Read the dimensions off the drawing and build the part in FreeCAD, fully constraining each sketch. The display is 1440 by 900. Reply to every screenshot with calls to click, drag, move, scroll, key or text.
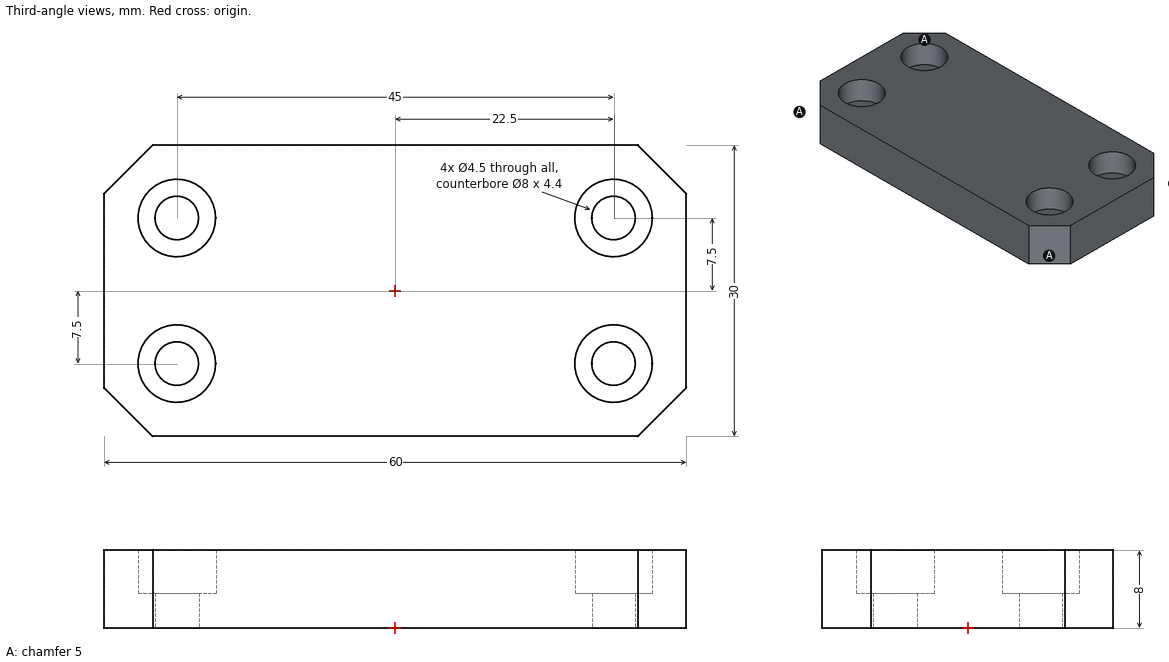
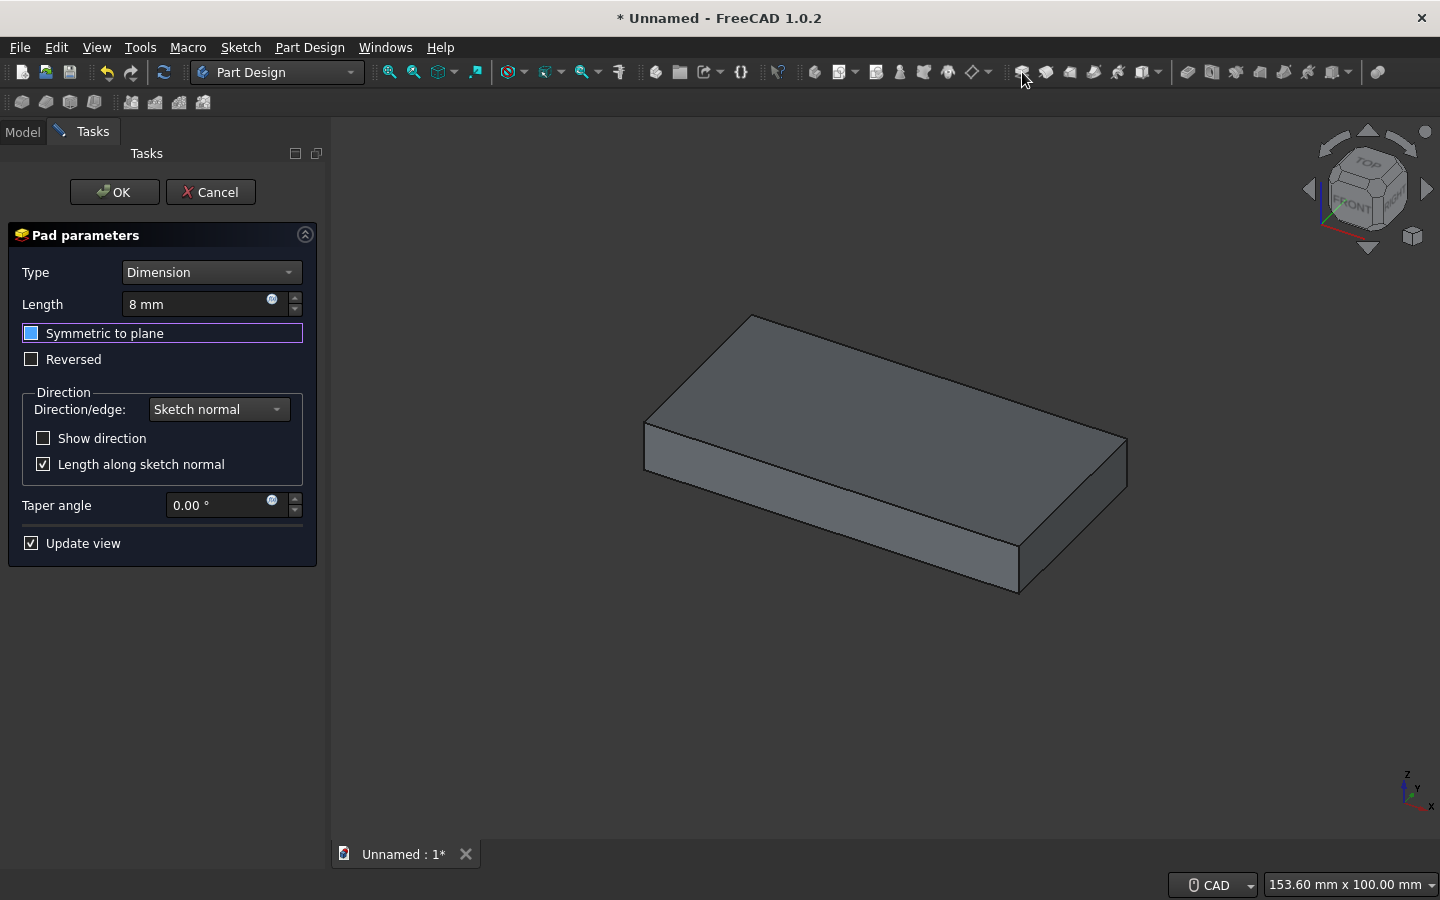
click(115, 192)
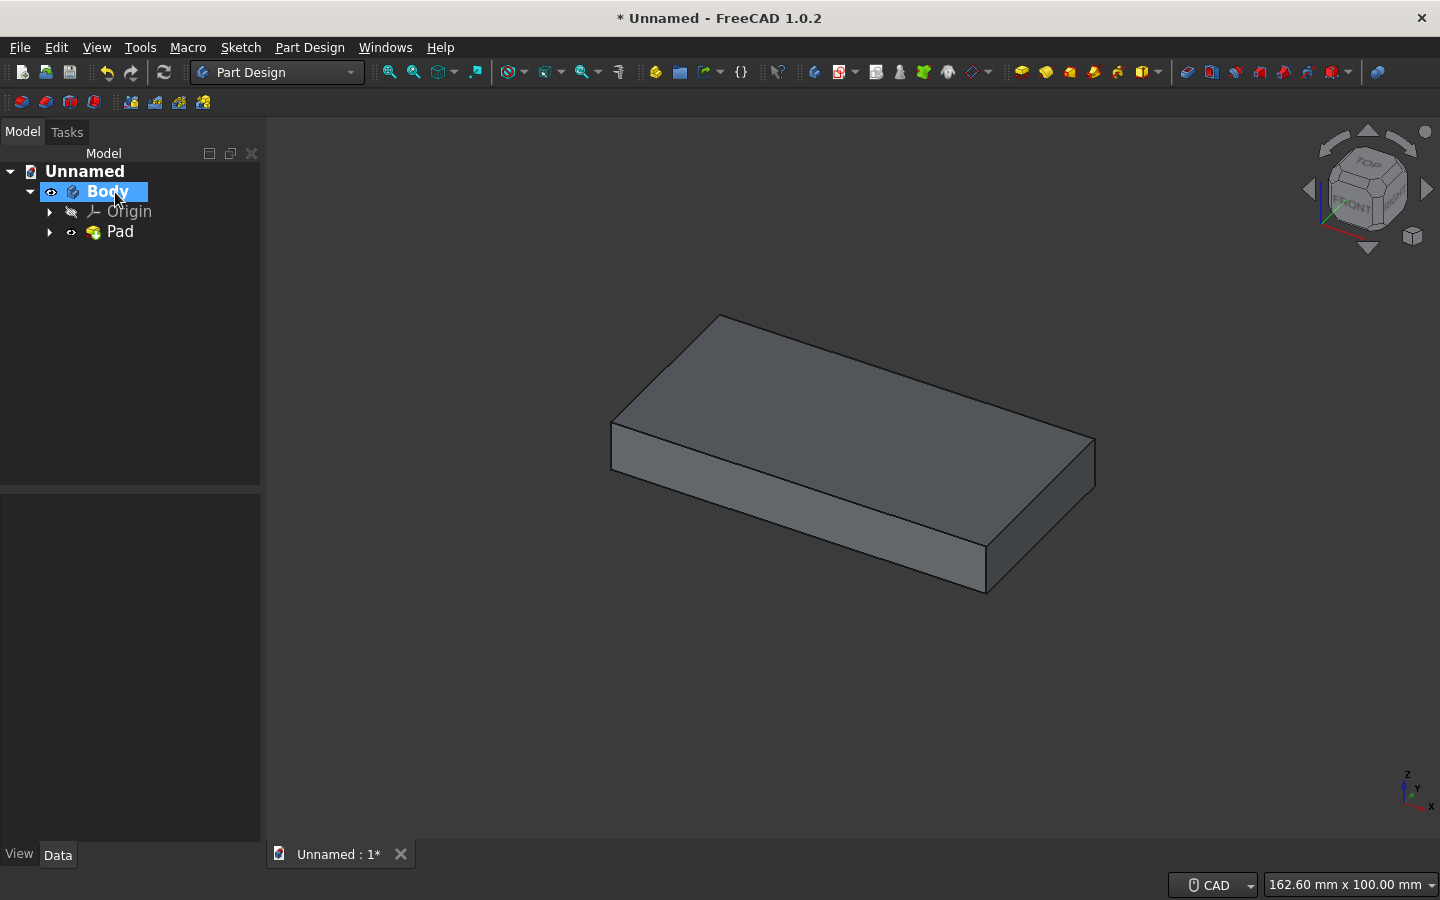
click(390, 72)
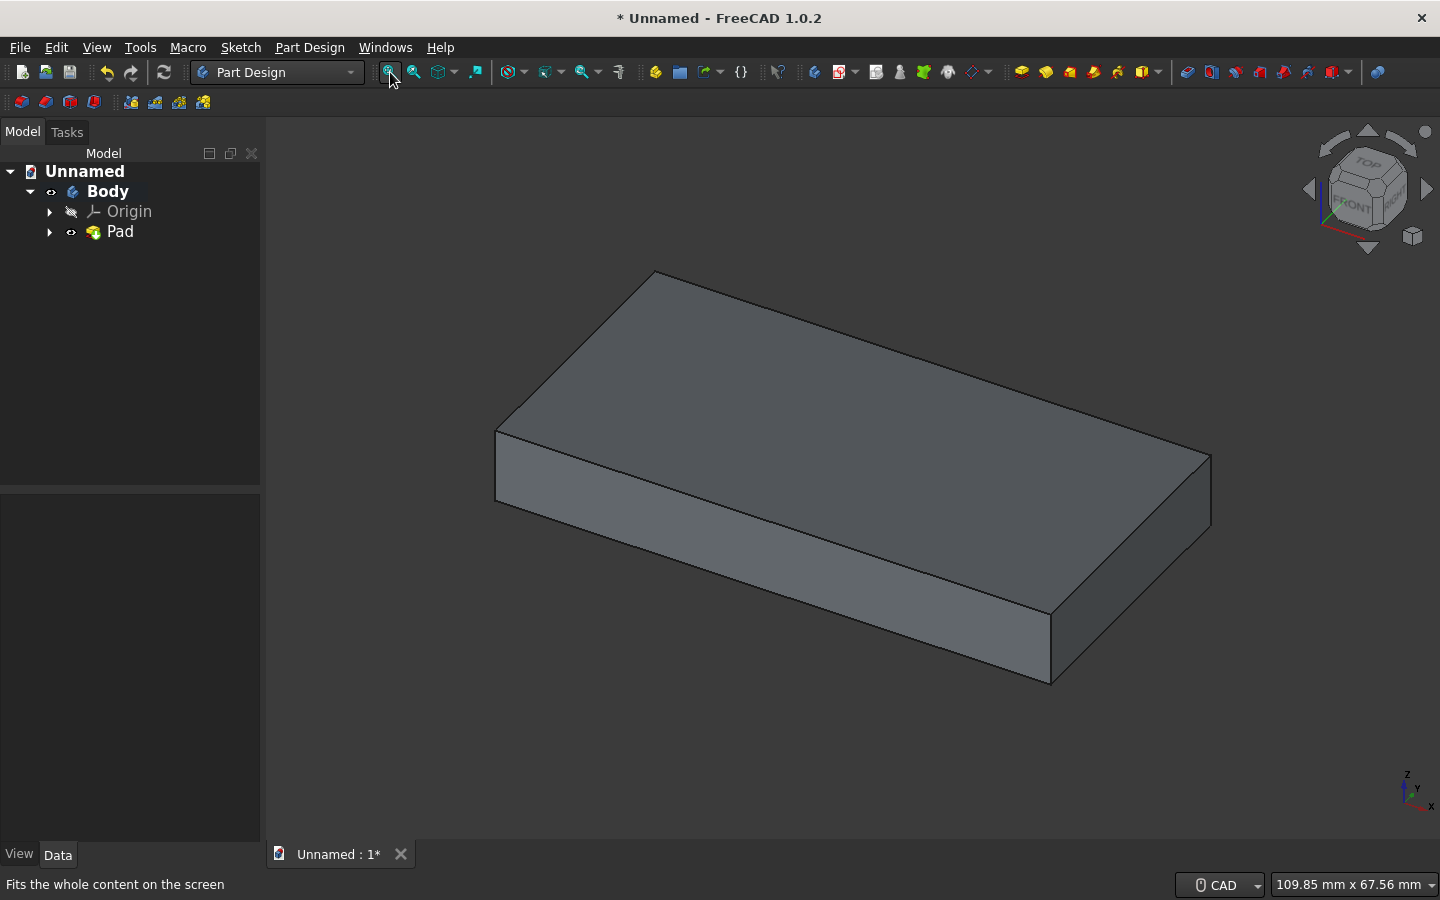
click(932, 468)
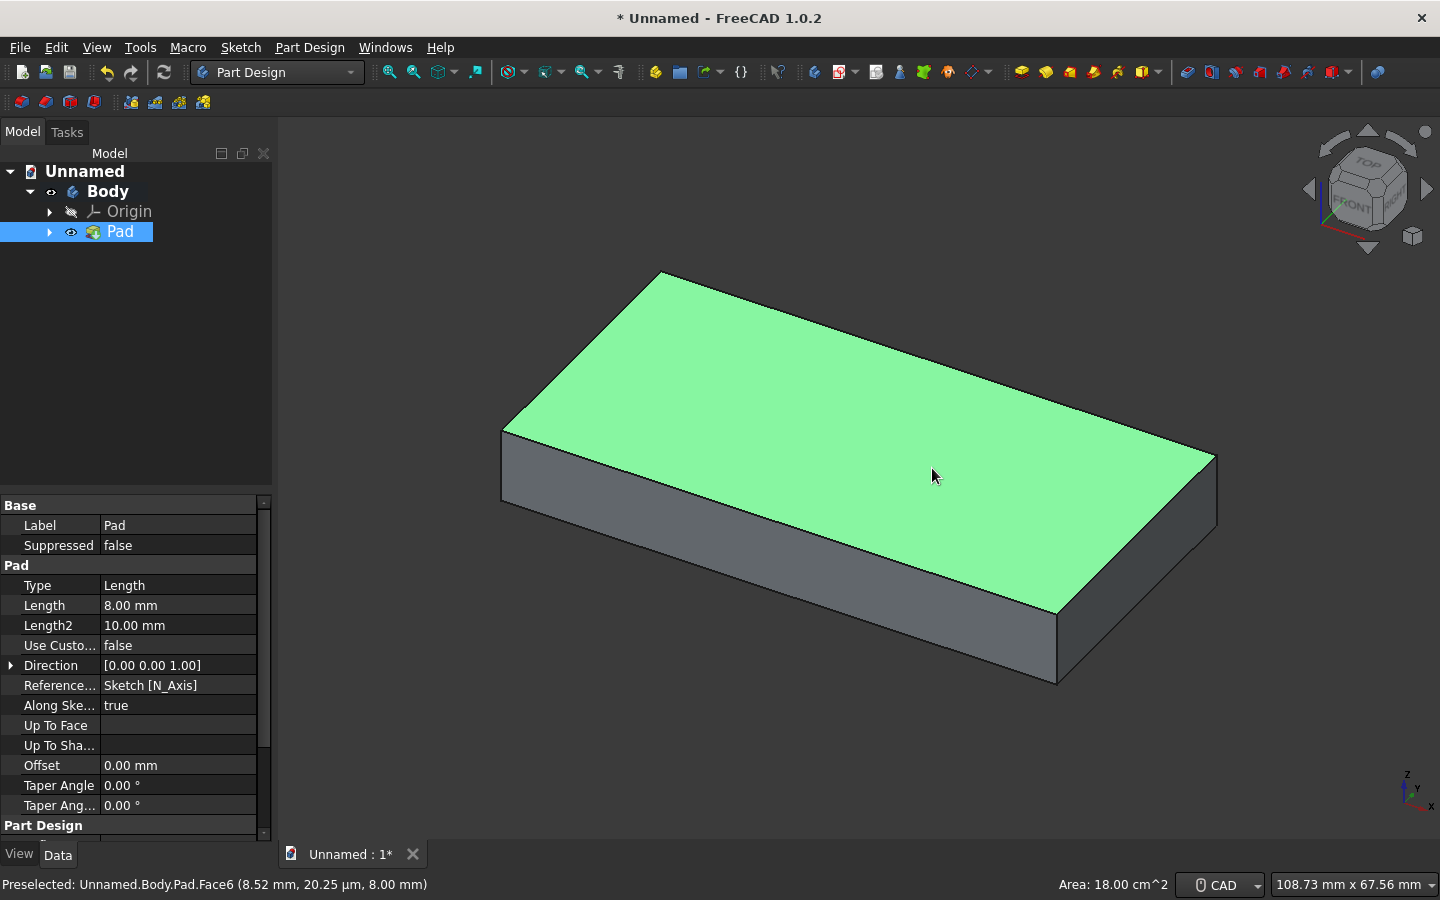
click(840, 72)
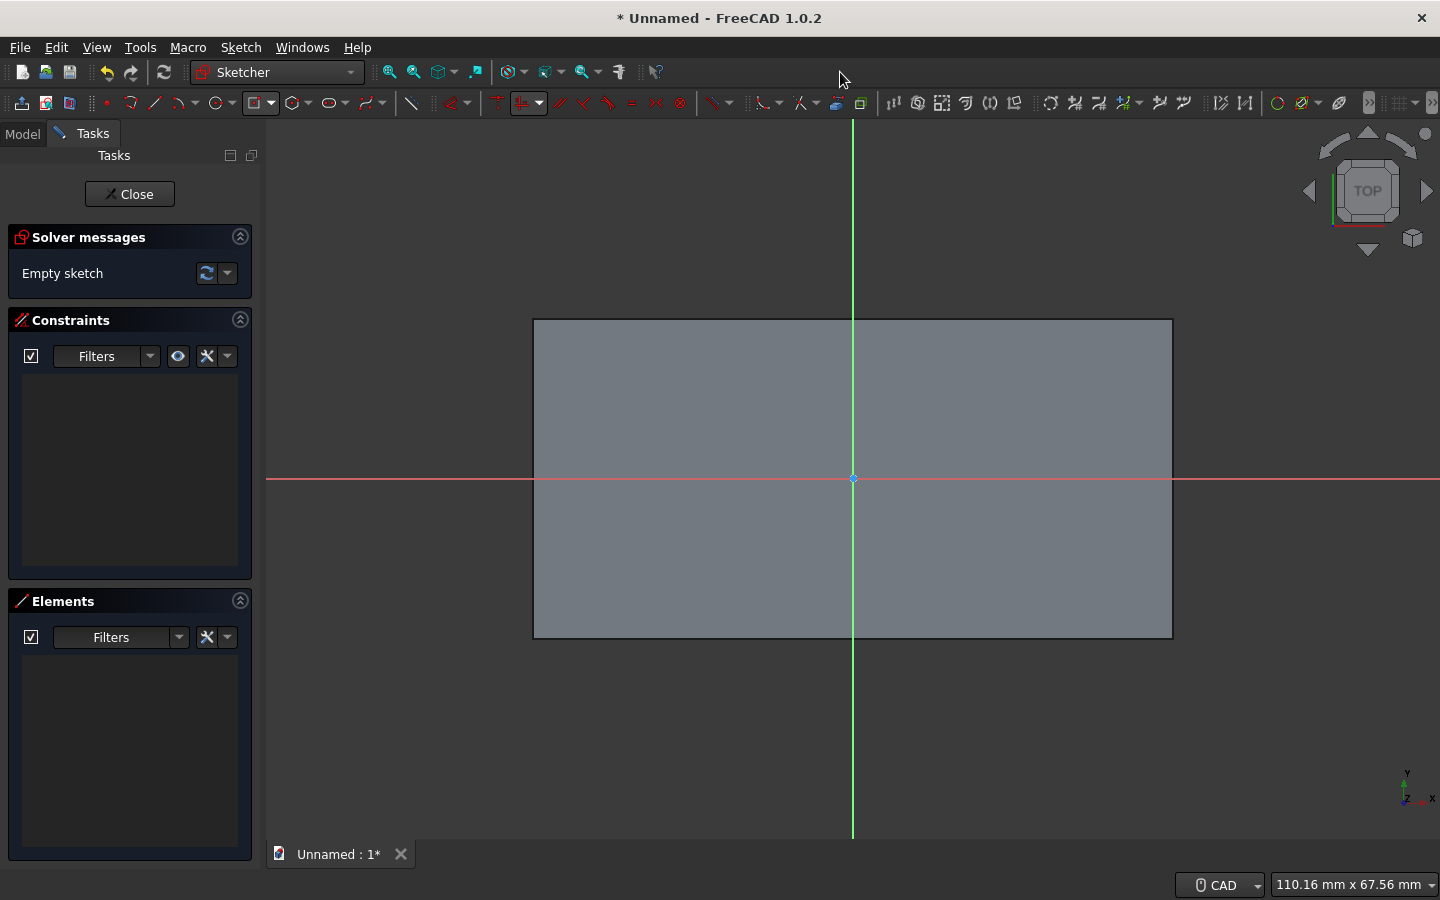
click(216, 104)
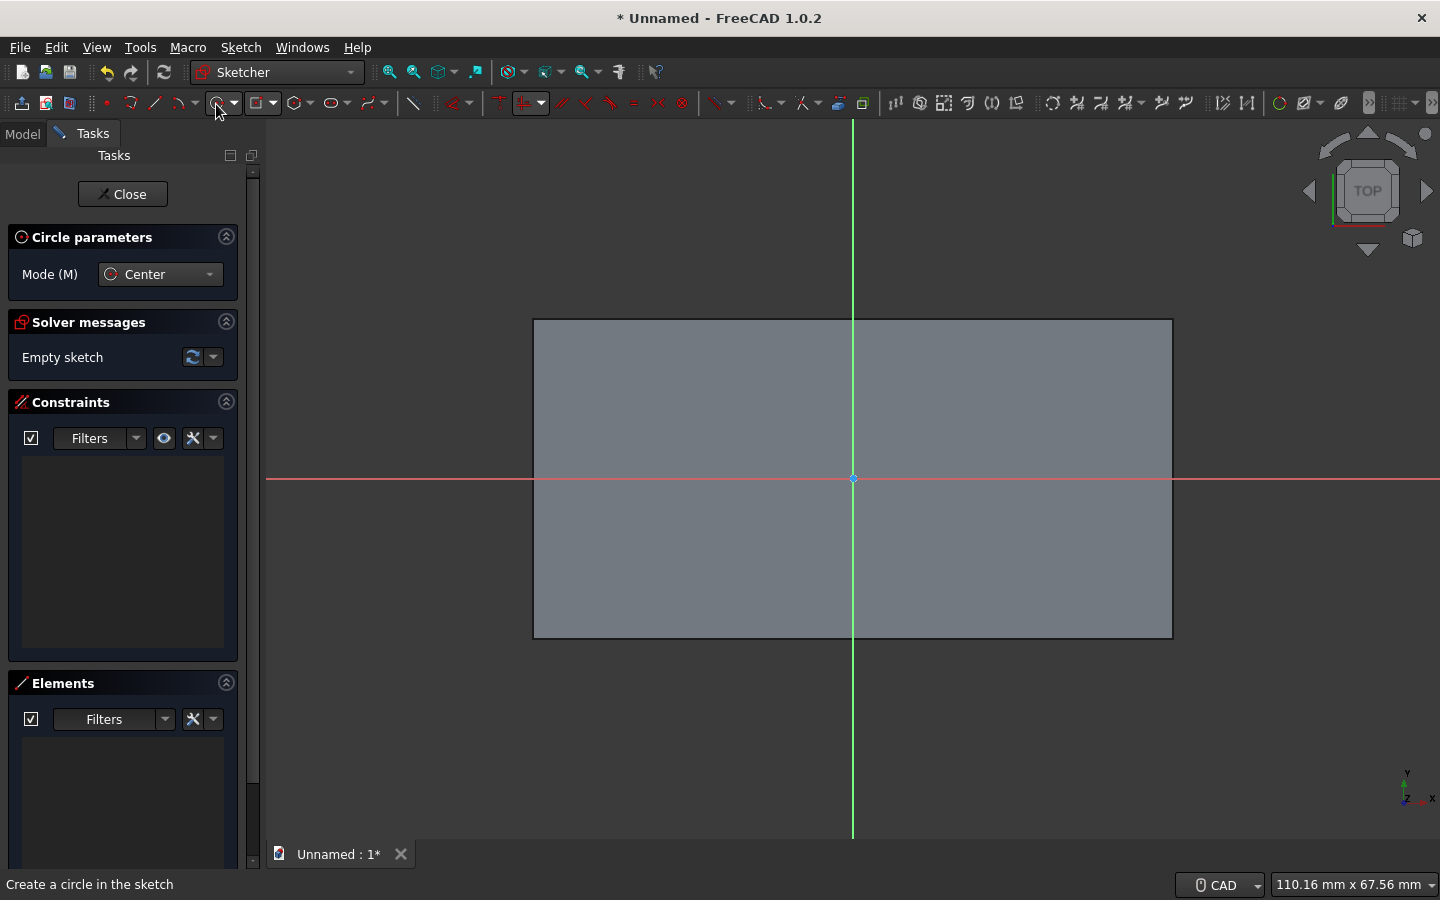
click(1093, 399)
click(1110, 382)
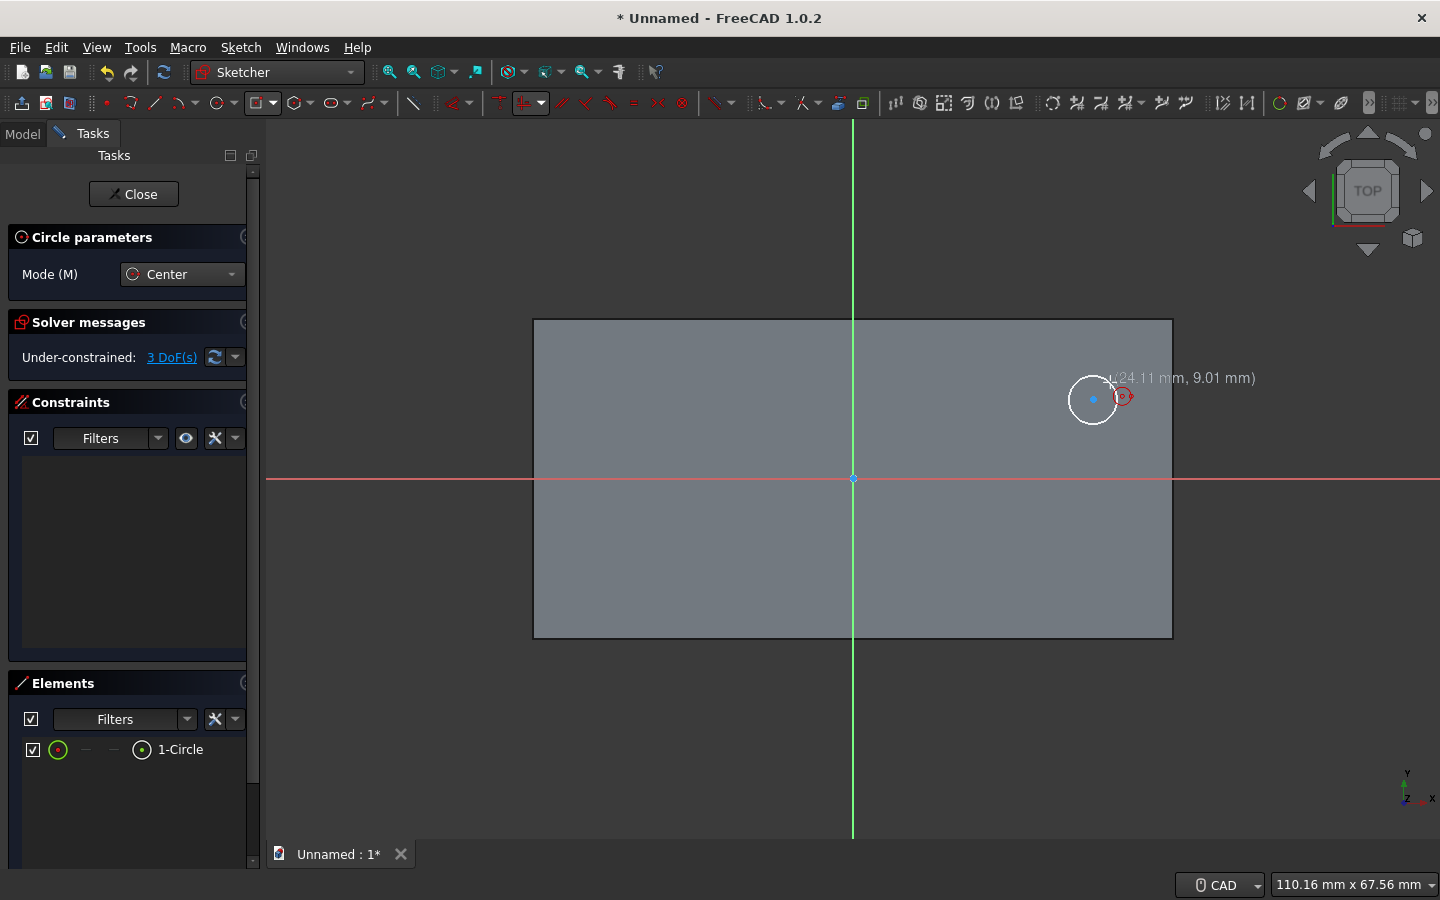
click(613, 399)
click(630, 382)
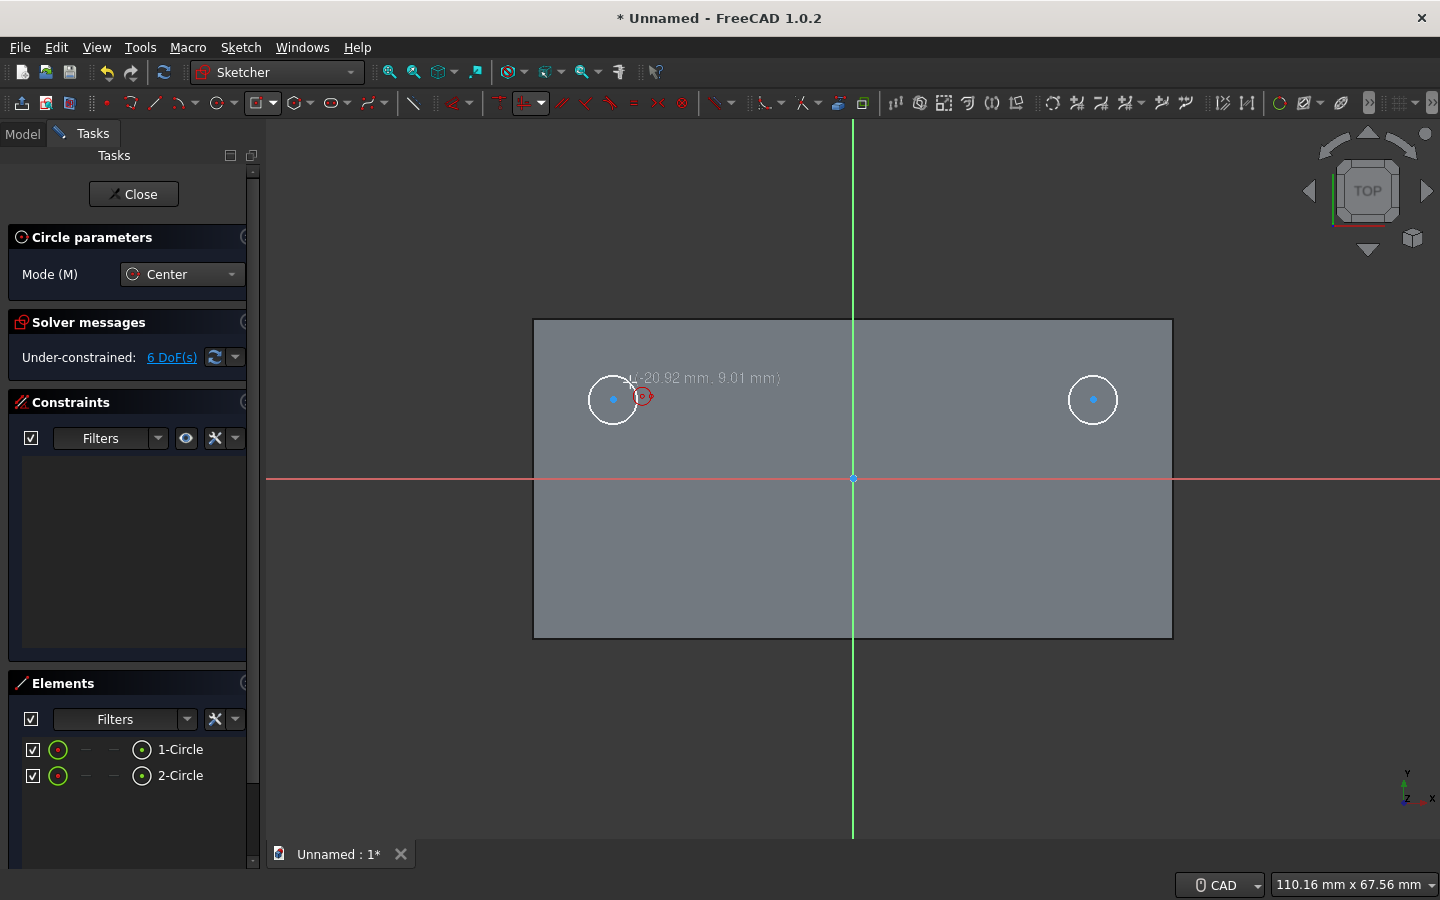
click(613, 559)
click(630, 542)